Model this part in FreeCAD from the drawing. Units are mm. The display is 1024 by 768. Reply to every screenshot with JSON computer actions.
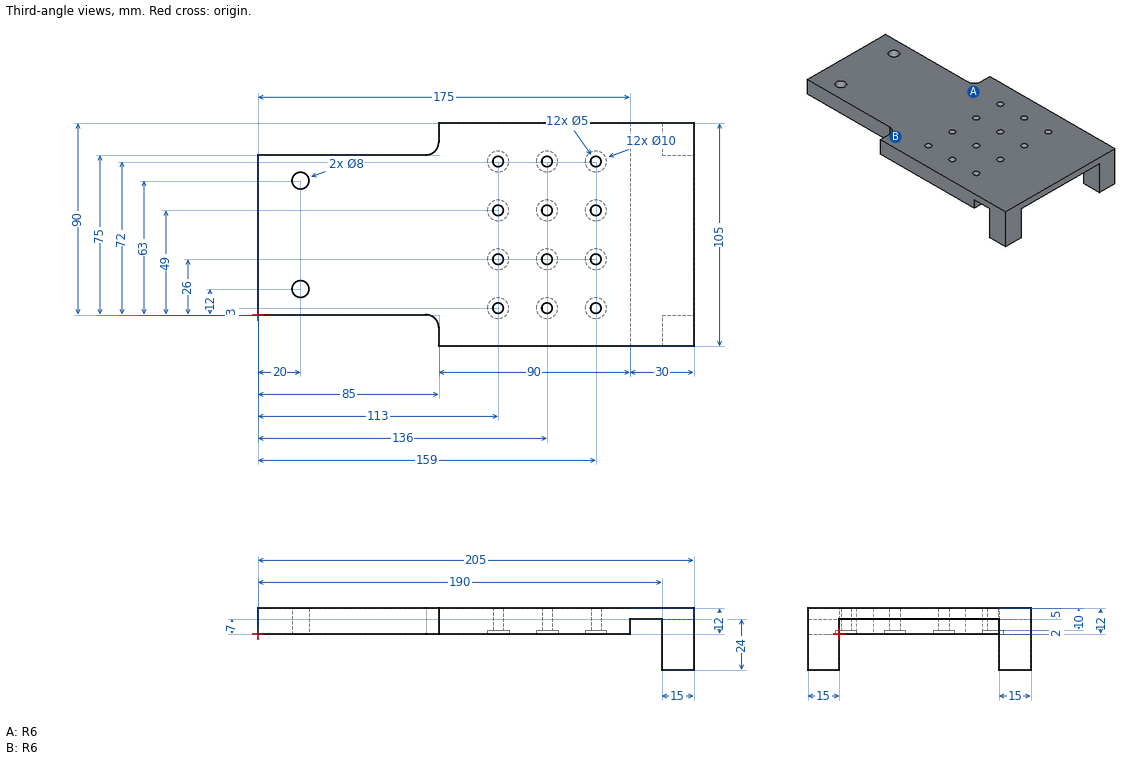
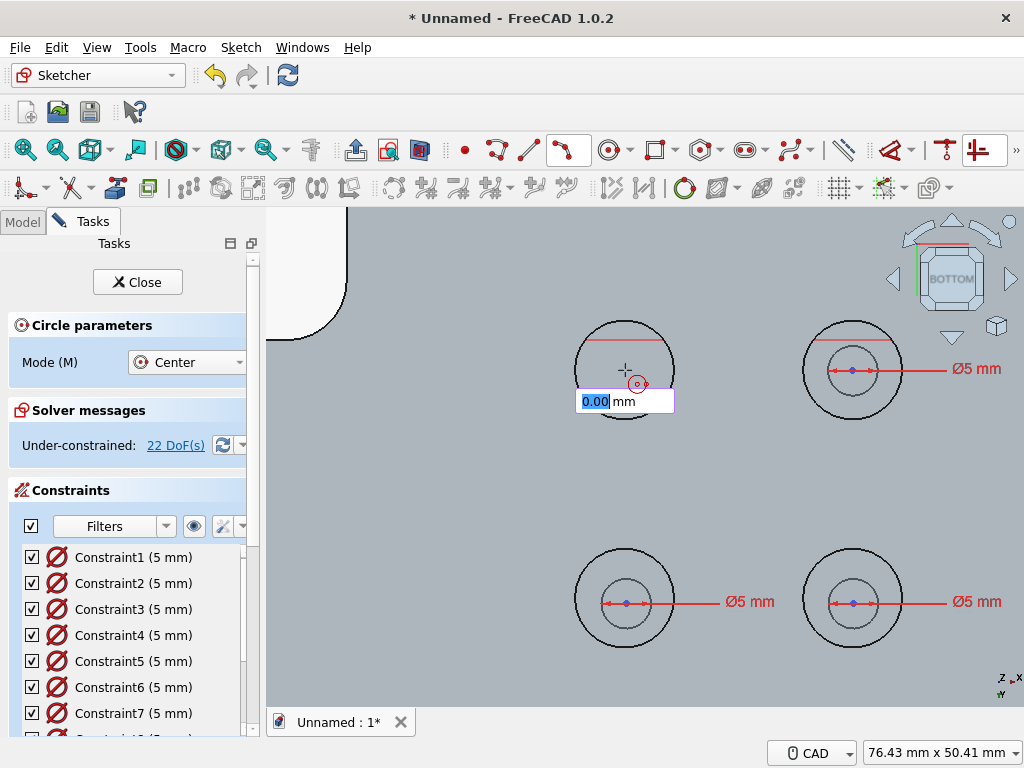
{"action": "scroll", "coordinate": [665, 374], "scroll_direction": "down", "scroll_amount": 7}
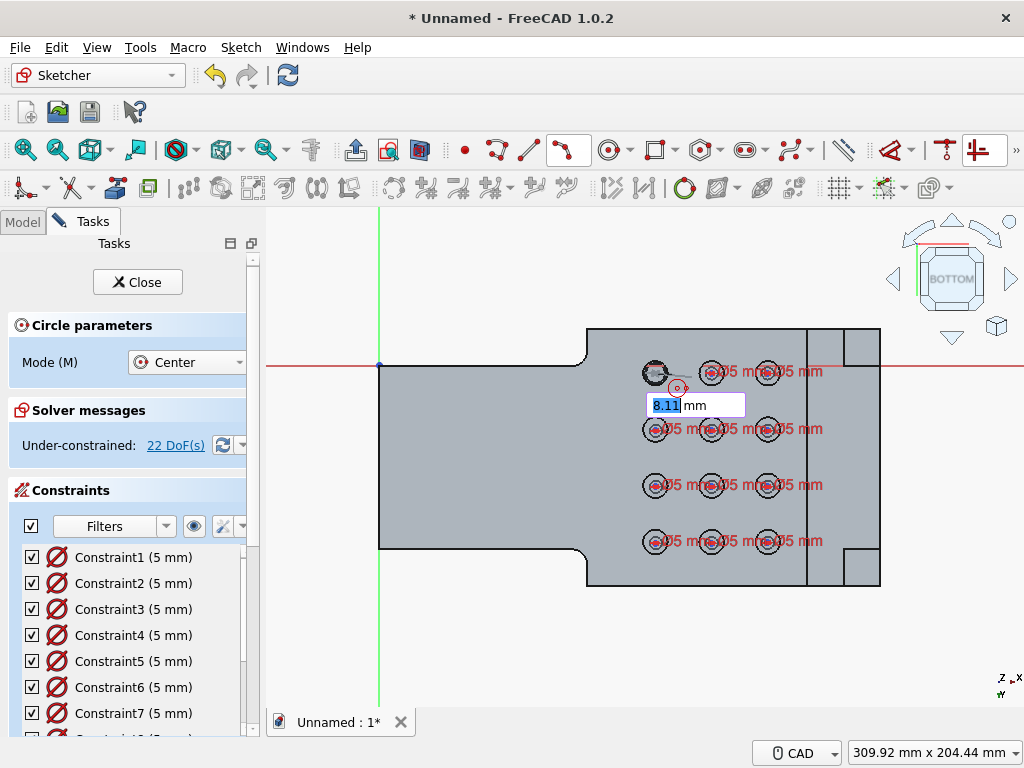
{"action": "scroll", "coordinate": [660, 378], "scroll_direction": "up", "scroll_amount": 2}
{"action": "mouse_move", "coordinate": [659, 377]}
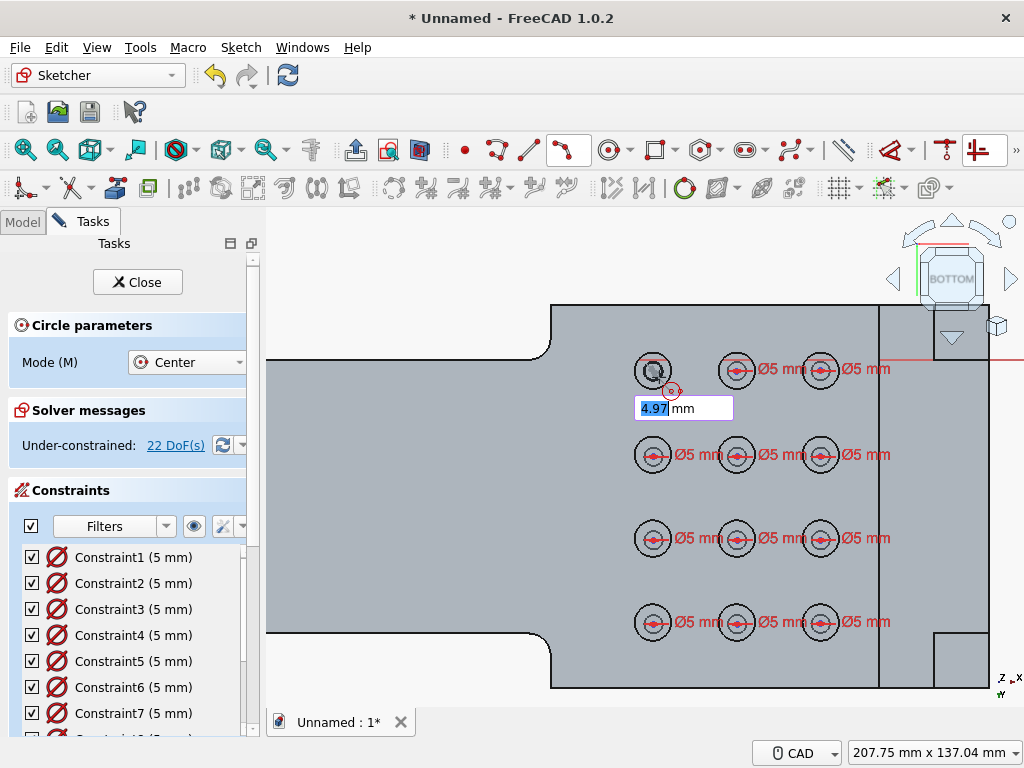
{"action": "type", "text": "5"}
{"action": "key", "text": "Return"}
{"action": "key", "text": "Escape"}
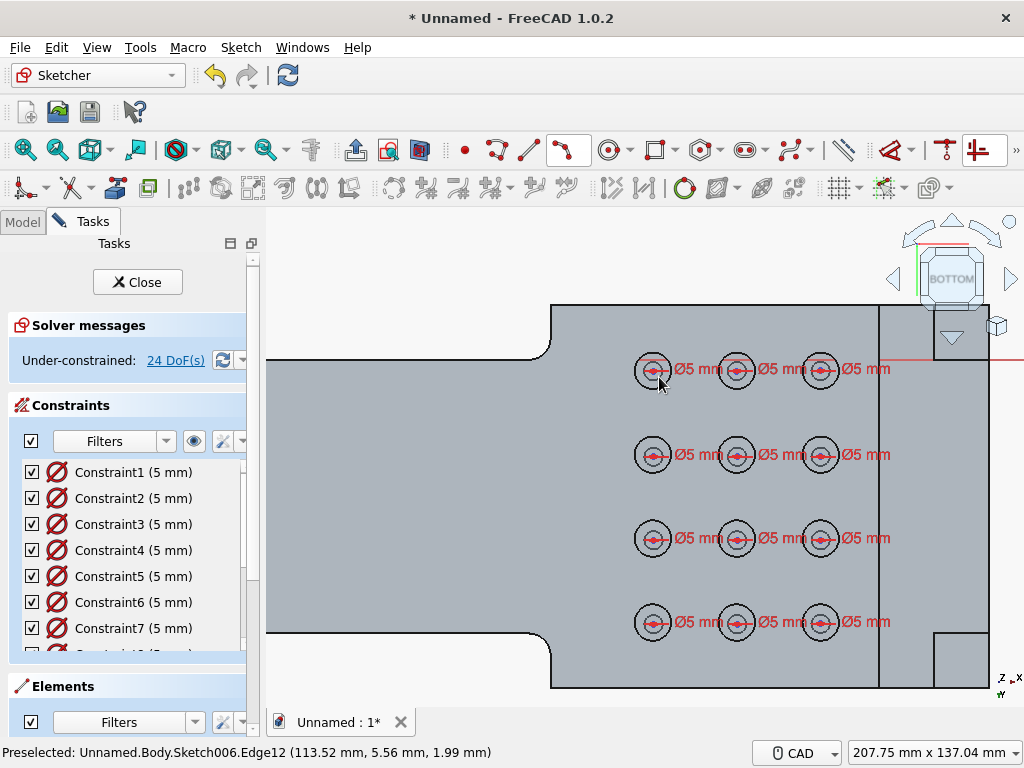
{"action": "left_click", "coordinate": [821, 624]}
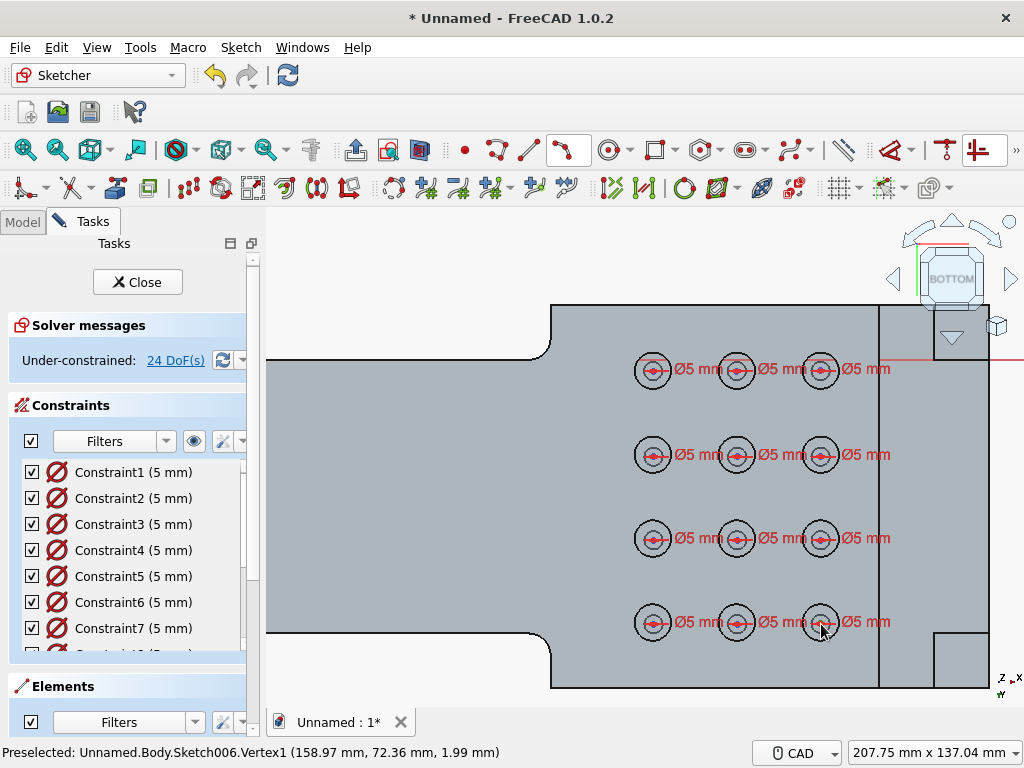
{"action": "left_click", "coordinate": [737, 624]}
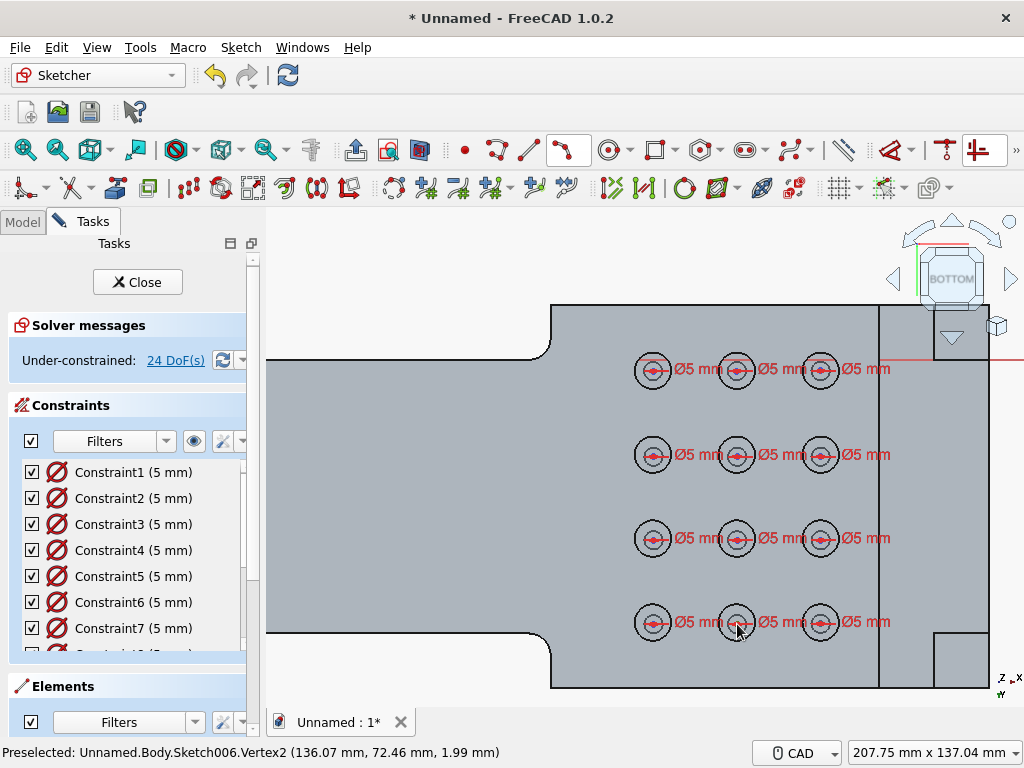
{"action": "key", "text": "h"}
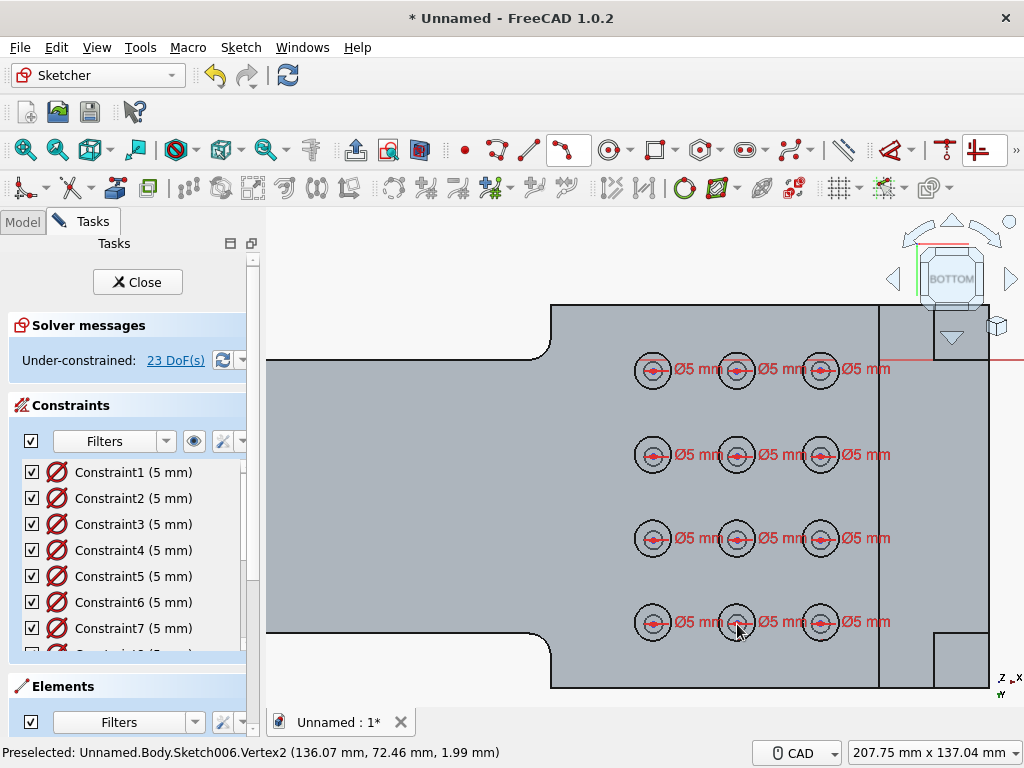
{"action": "left_click", "coordinate": [737, 624]}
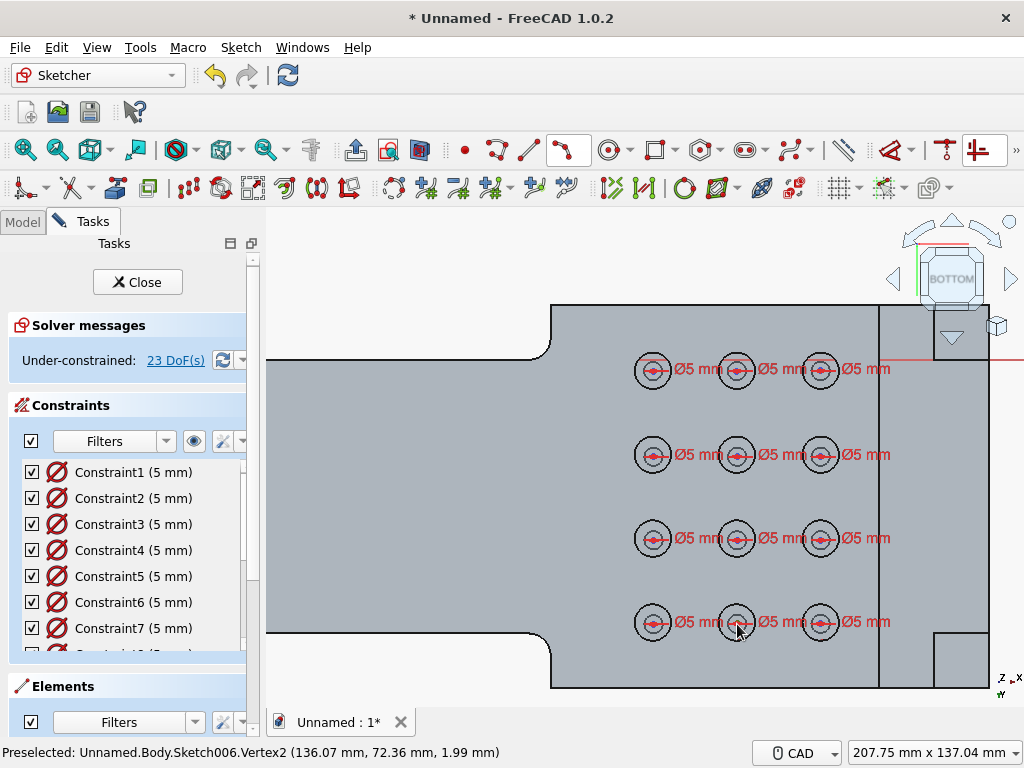
{"action": "left_click", "coordinate": [654, 624]}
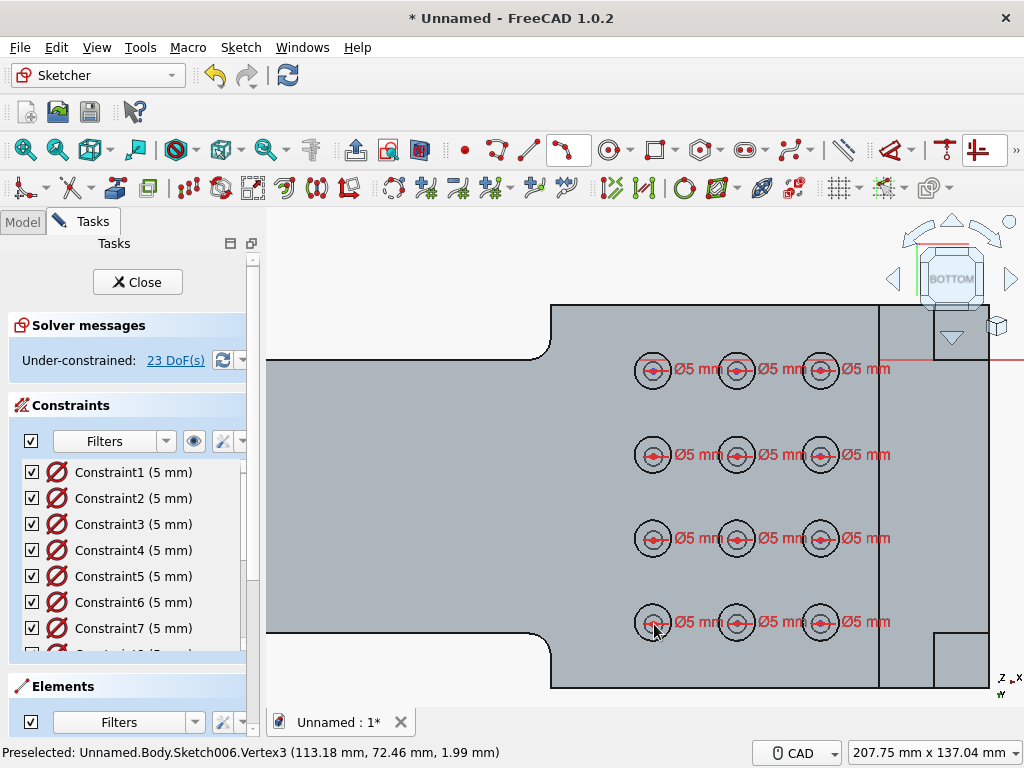
{"action": "key", "text": "h"}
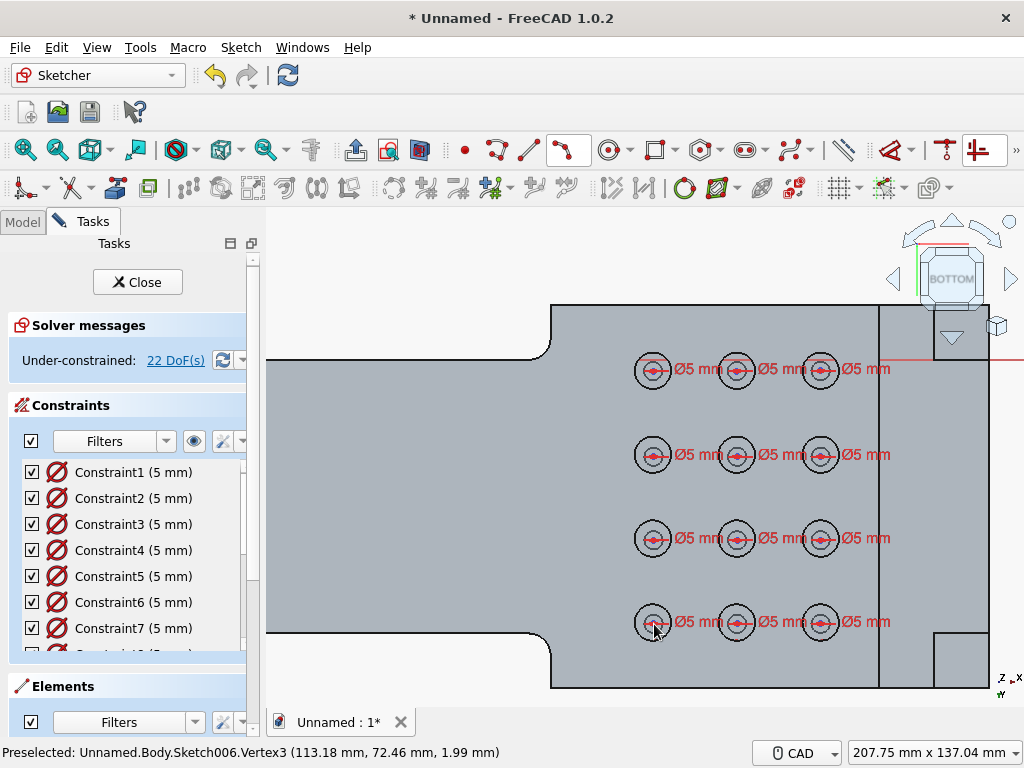
{"action": "left_click", "coordinate": [654, 624]}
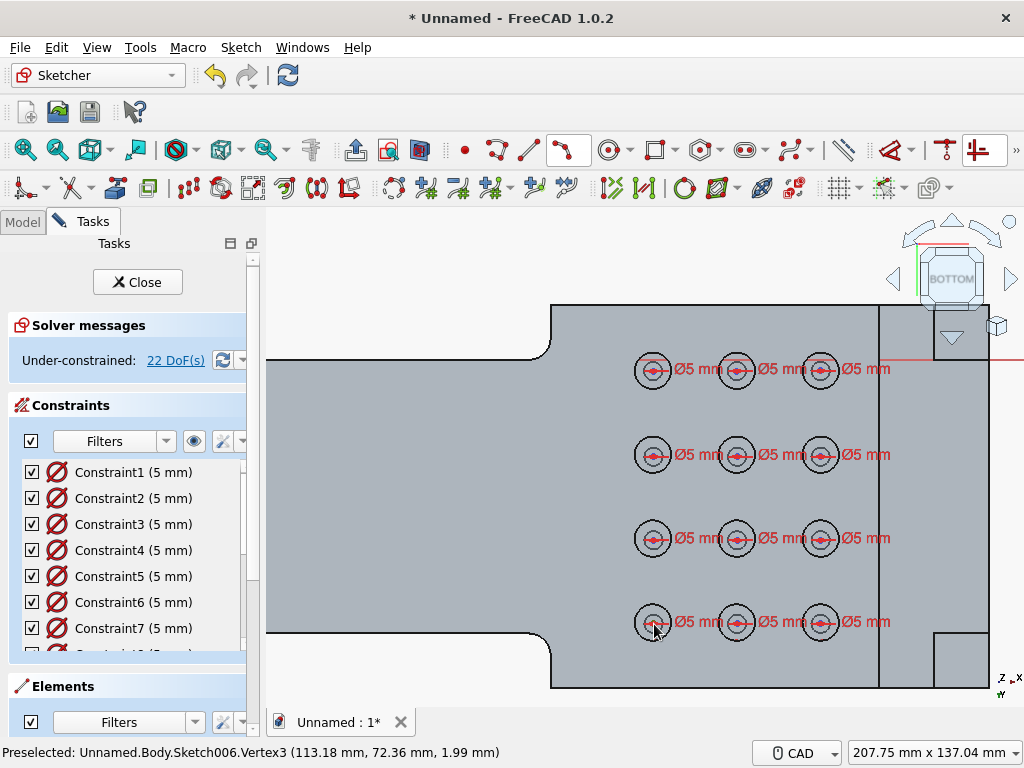
{"action": "left_click", "coordinate": [654, 540]}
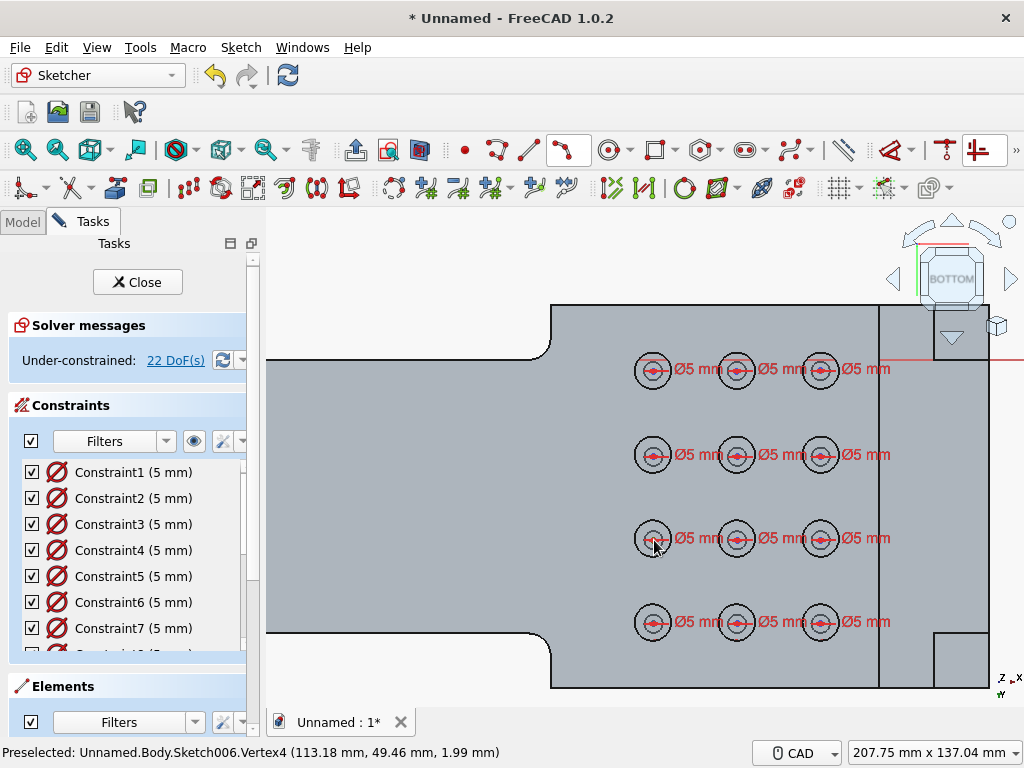
{"action": "key", "text": "v"}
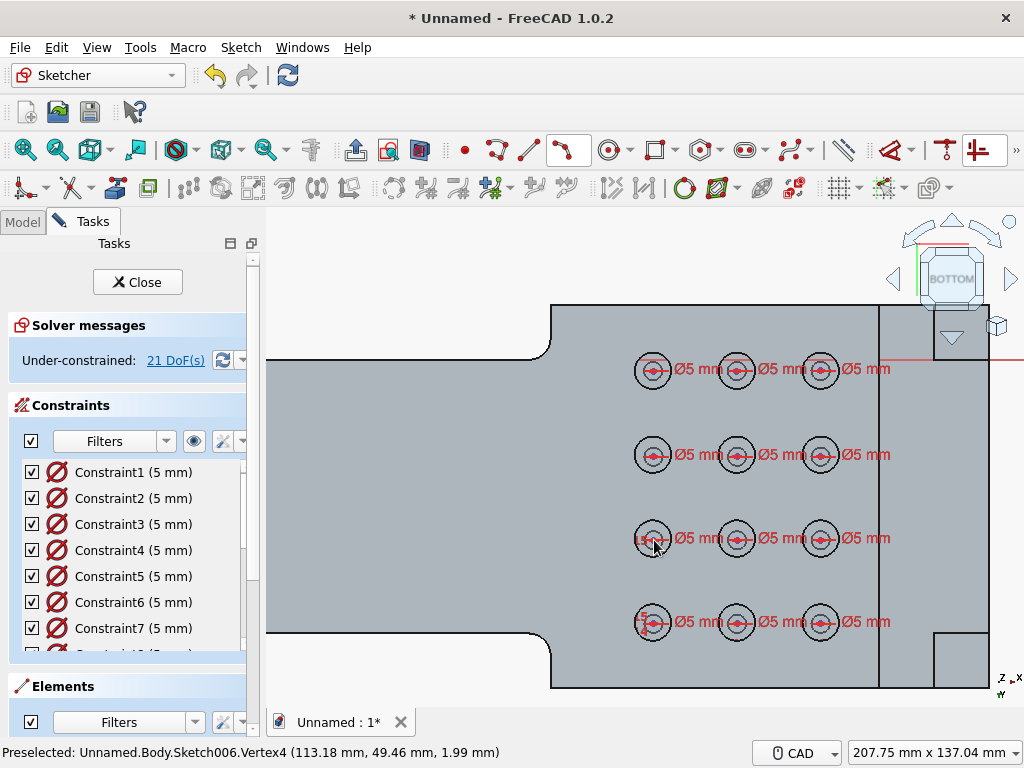
{"action": "left_click", "coordinate": [737, 624]}